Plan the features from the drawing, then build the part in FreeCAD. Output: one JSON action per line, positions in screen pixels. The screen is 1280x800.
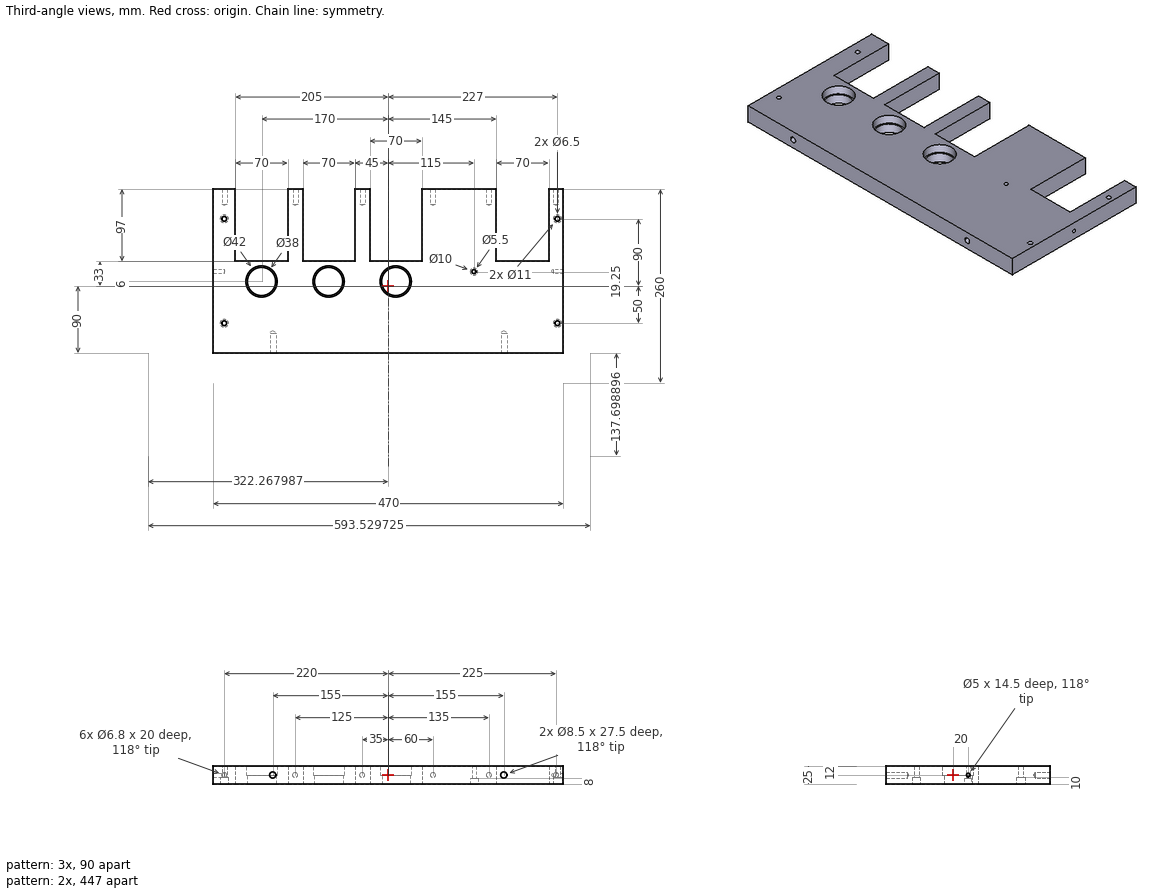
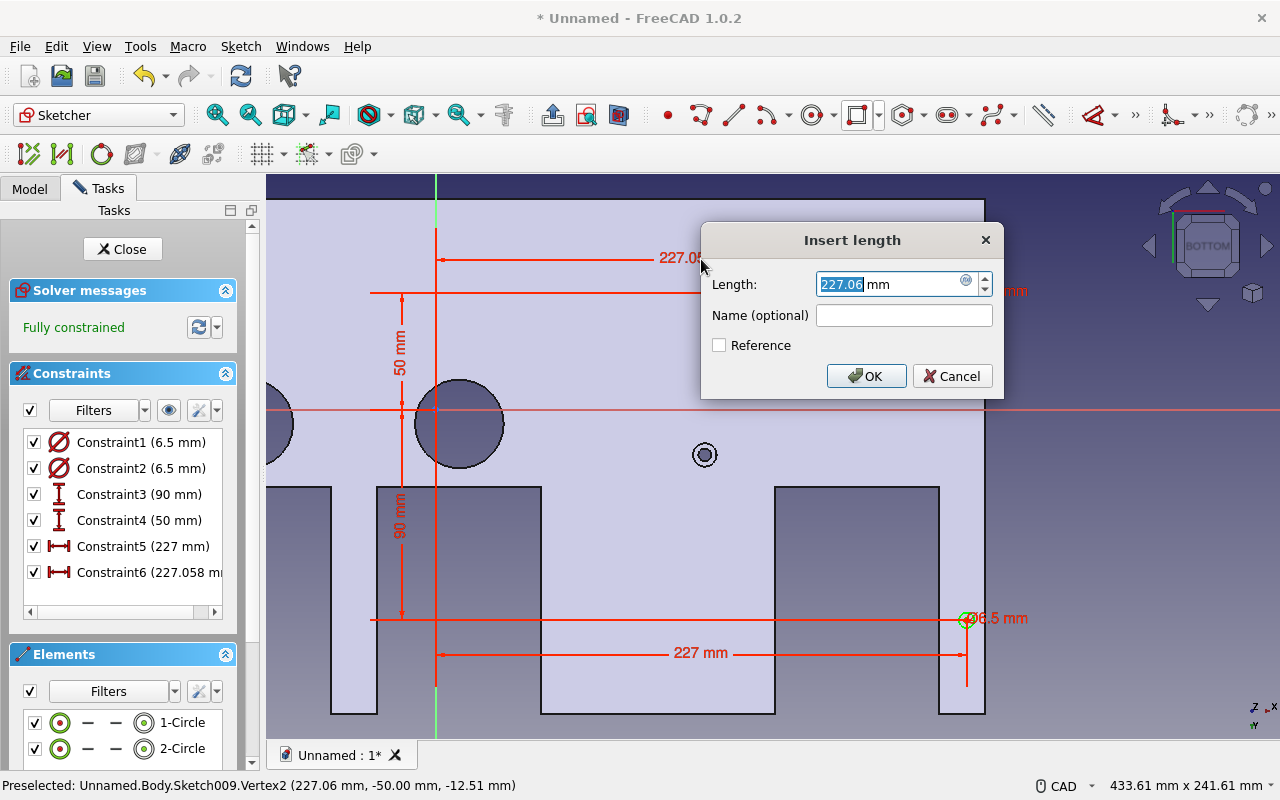
{"action": "type", "text": "227"}
{"action": "key", "text": "Return"}
{"action": "key", "text": "Escape"}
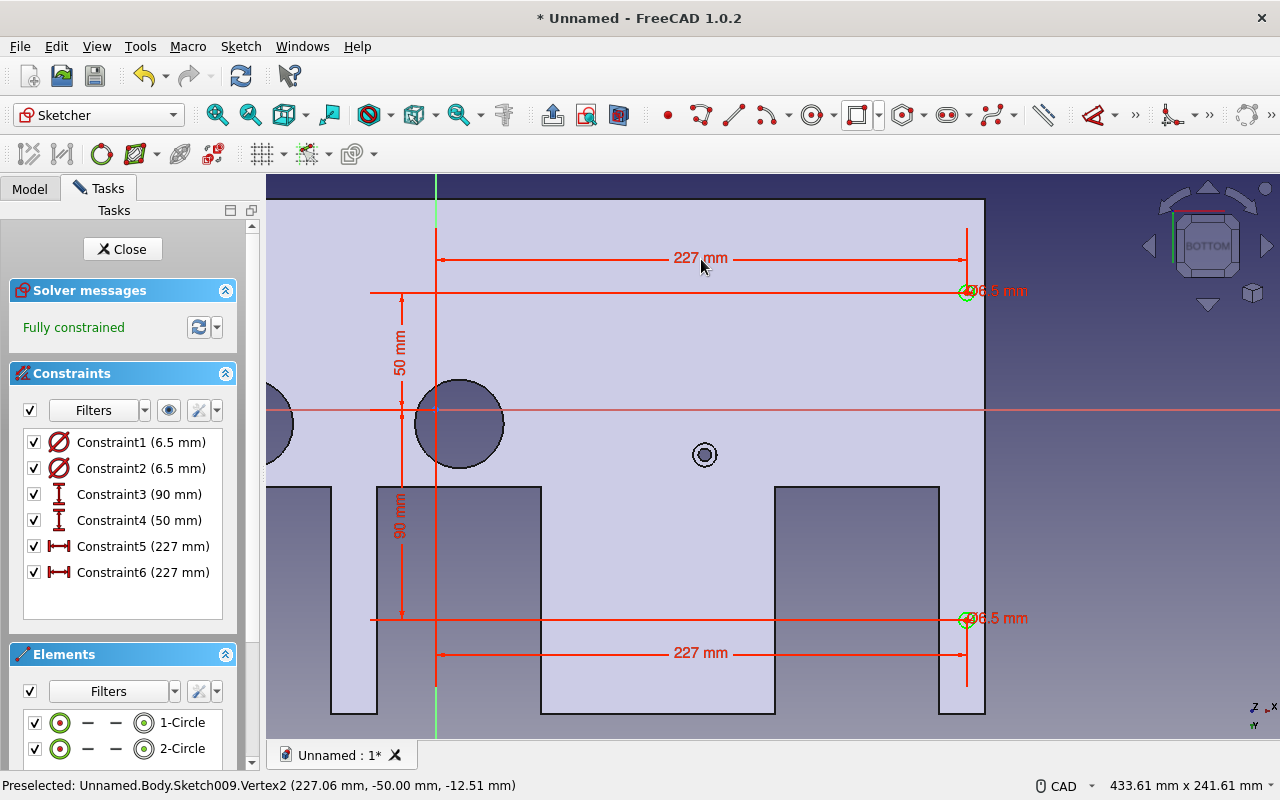
{"action": "left_click", "coordinate": [123, 249]}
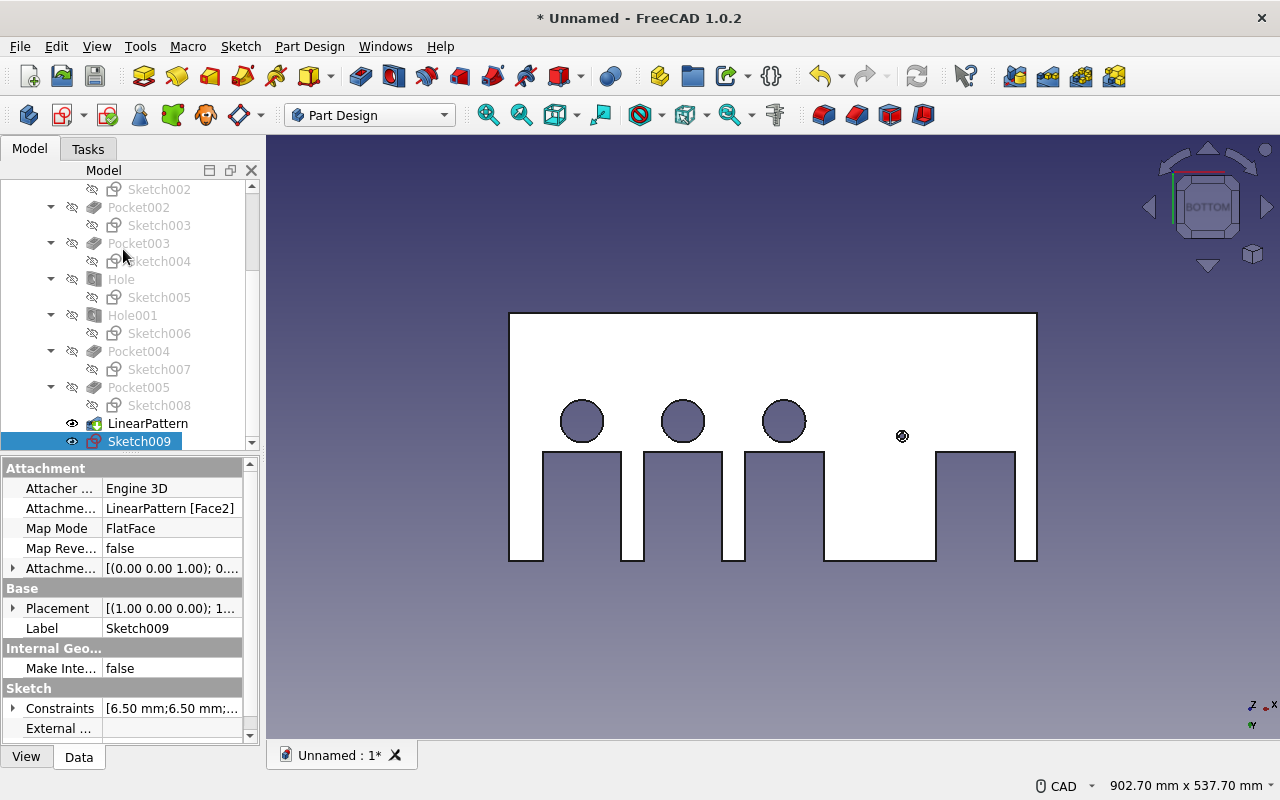
{"action": "left_click", "coordinate": [361, 76]}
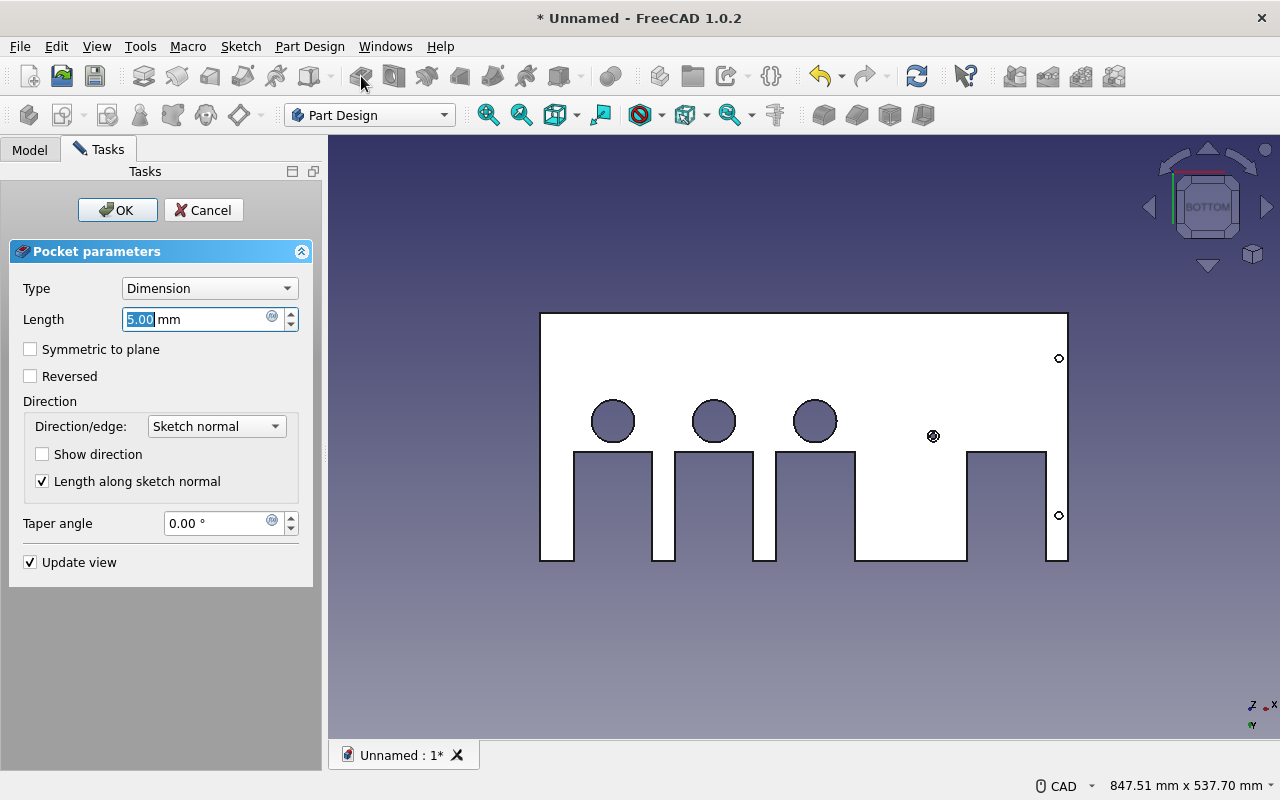
{"action": "left_click", "coordinate": [210, 288]}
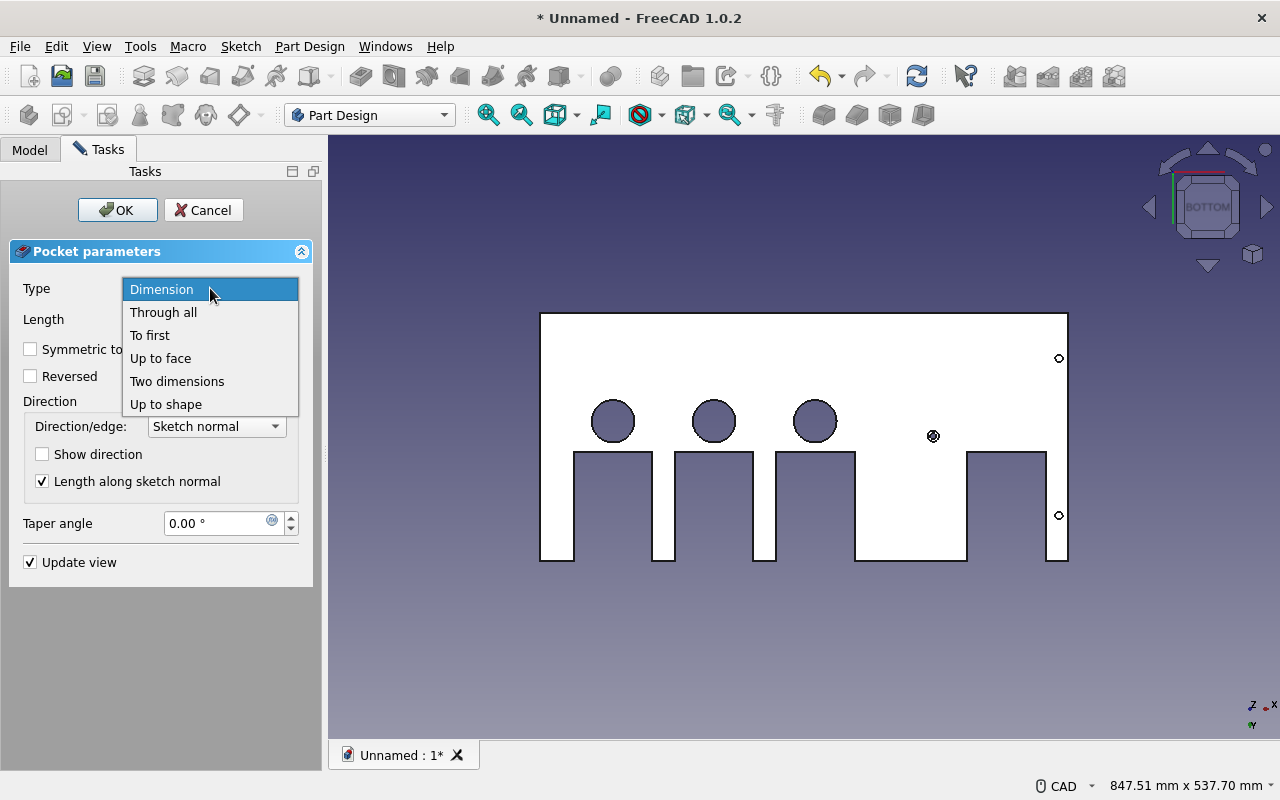
{"action": "left_click", "coordinate": [208, 312]}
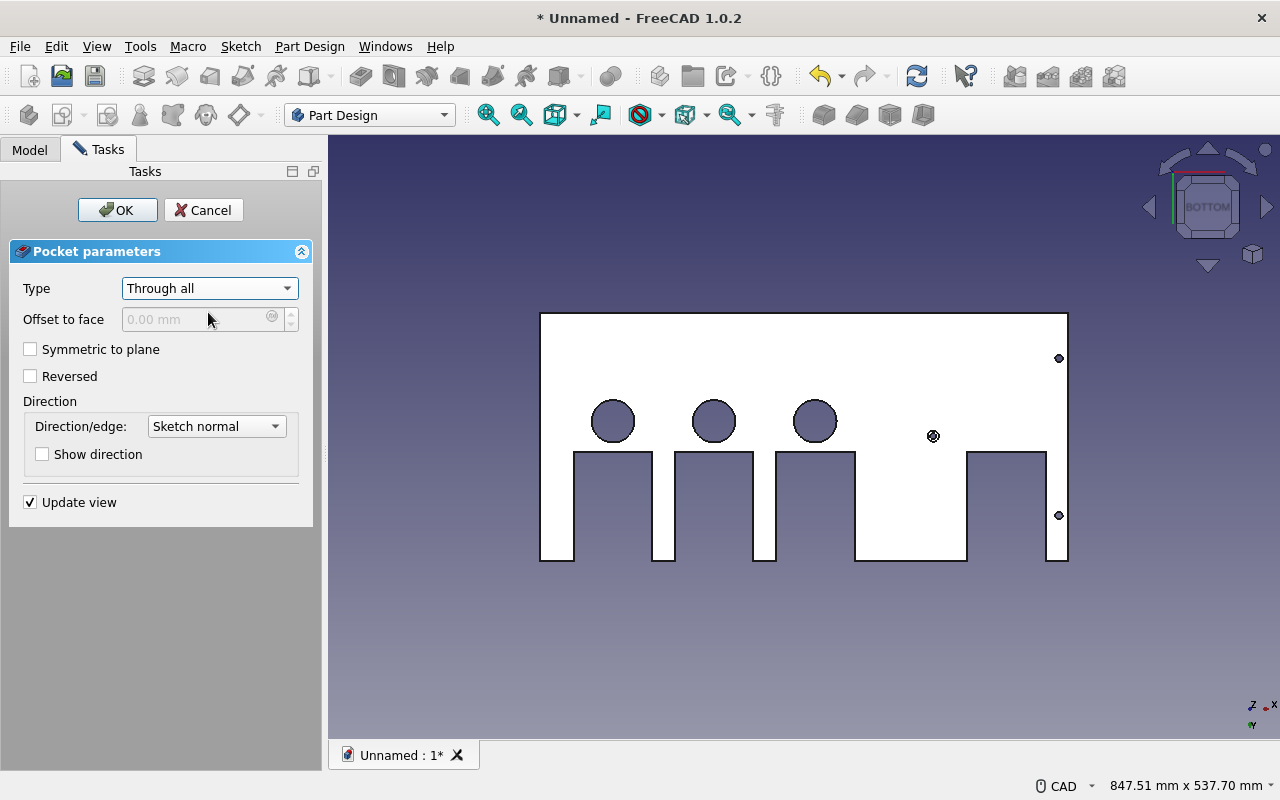
{"action": "left_click", "coordinate": [118, 210]}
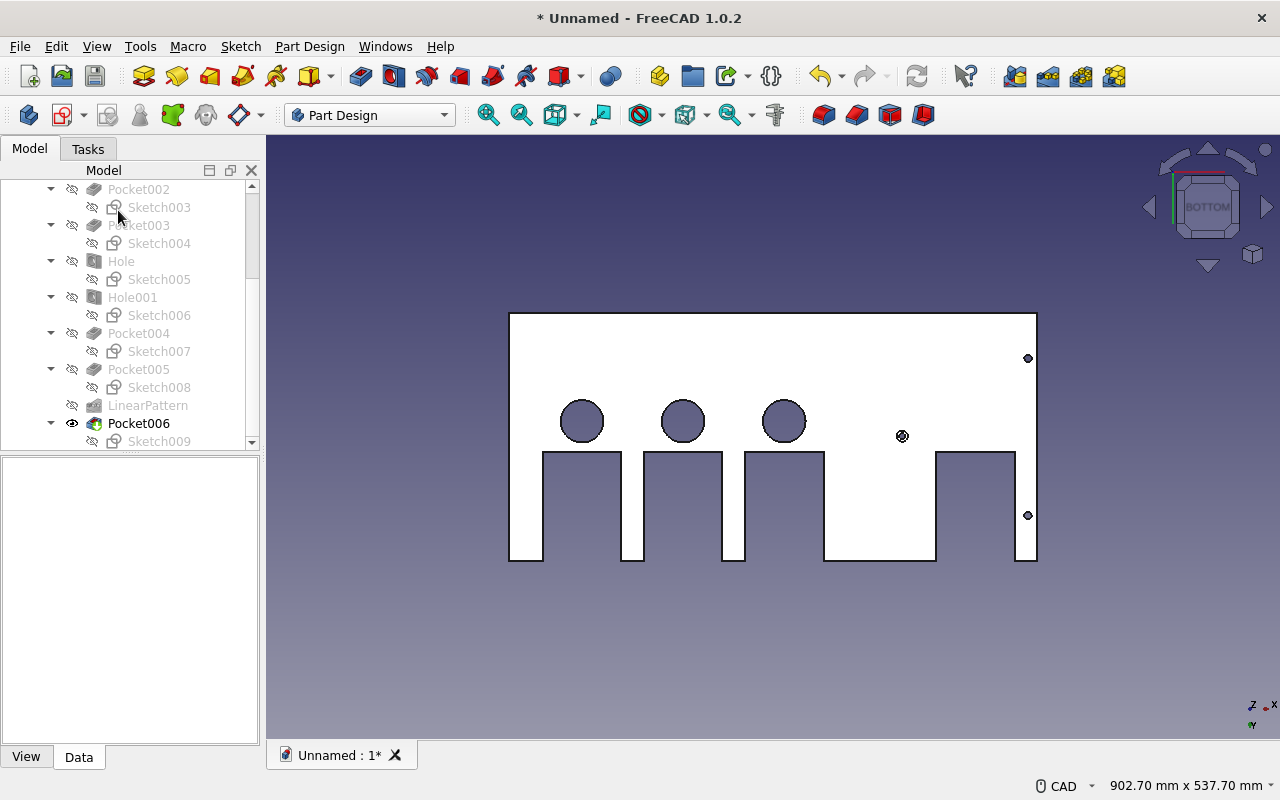
{"action": "left_click", "coordinate": [924, 365]}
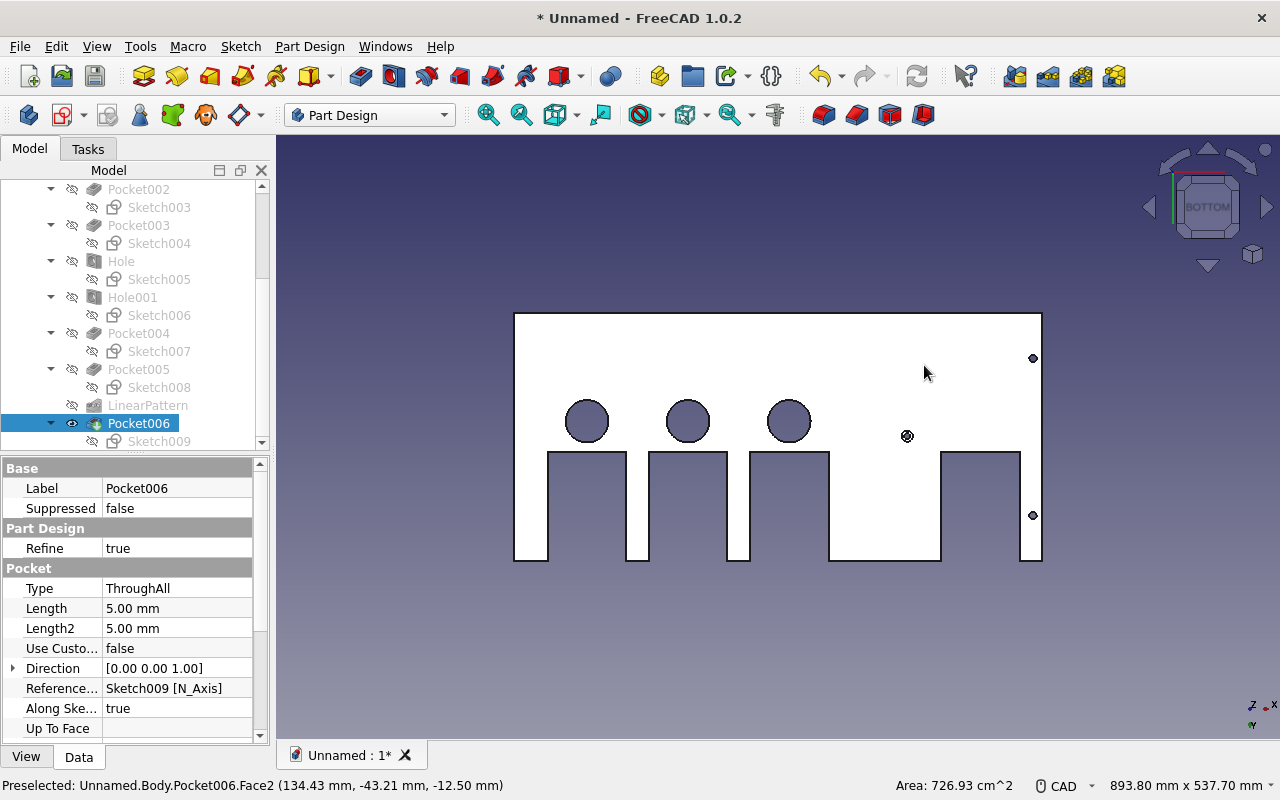
{"action": "left_click", "coordinate": [62, 116]}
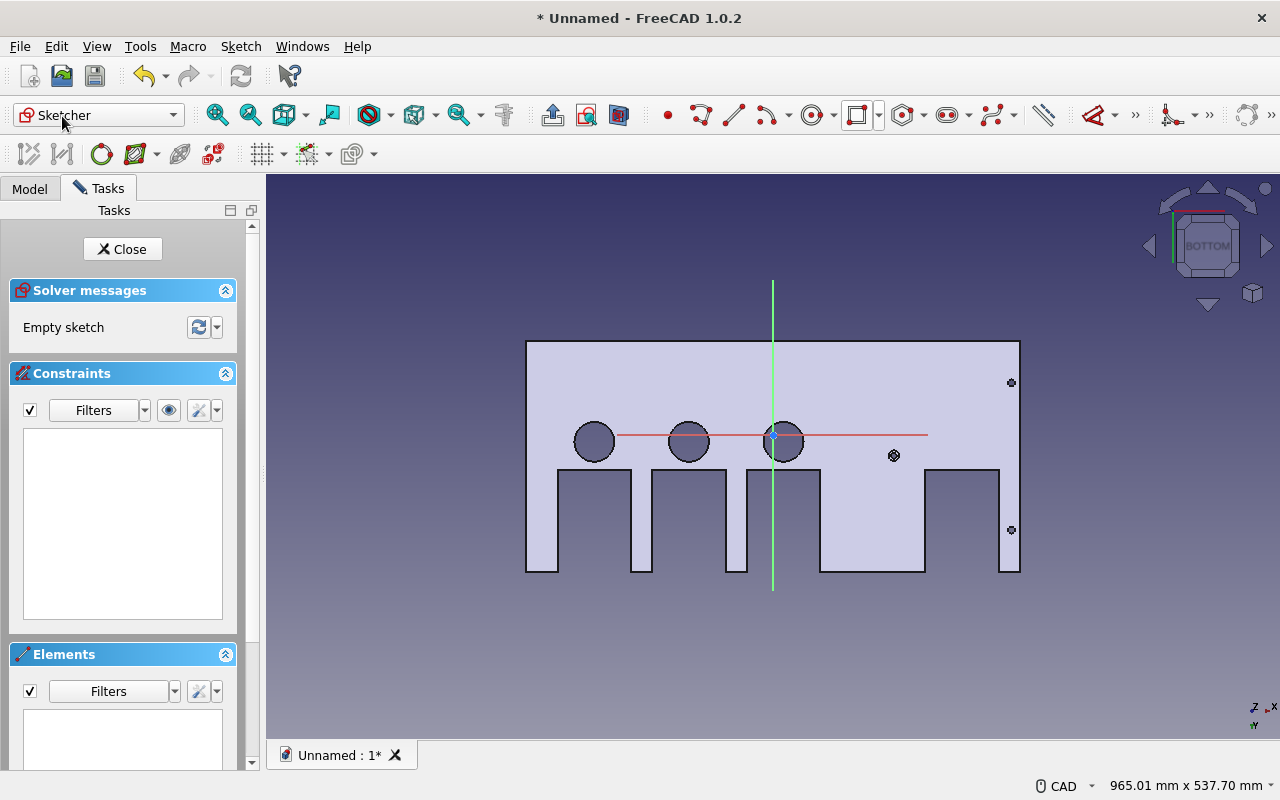
{"action": "scroll", "coordinate": [1051, 457], "scroll_direction": "up", "scroll_amount": 4}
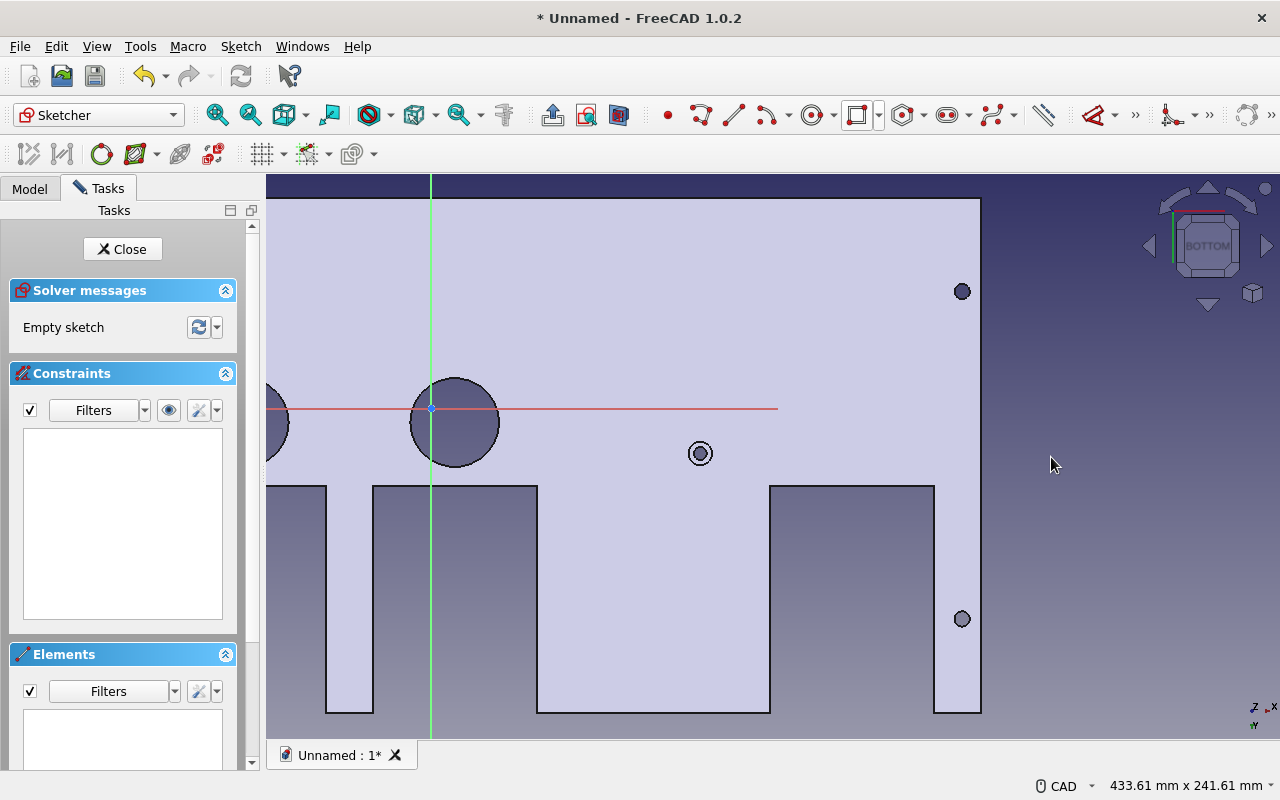
{"action": "left_click", "coordinate": [812, 116]}